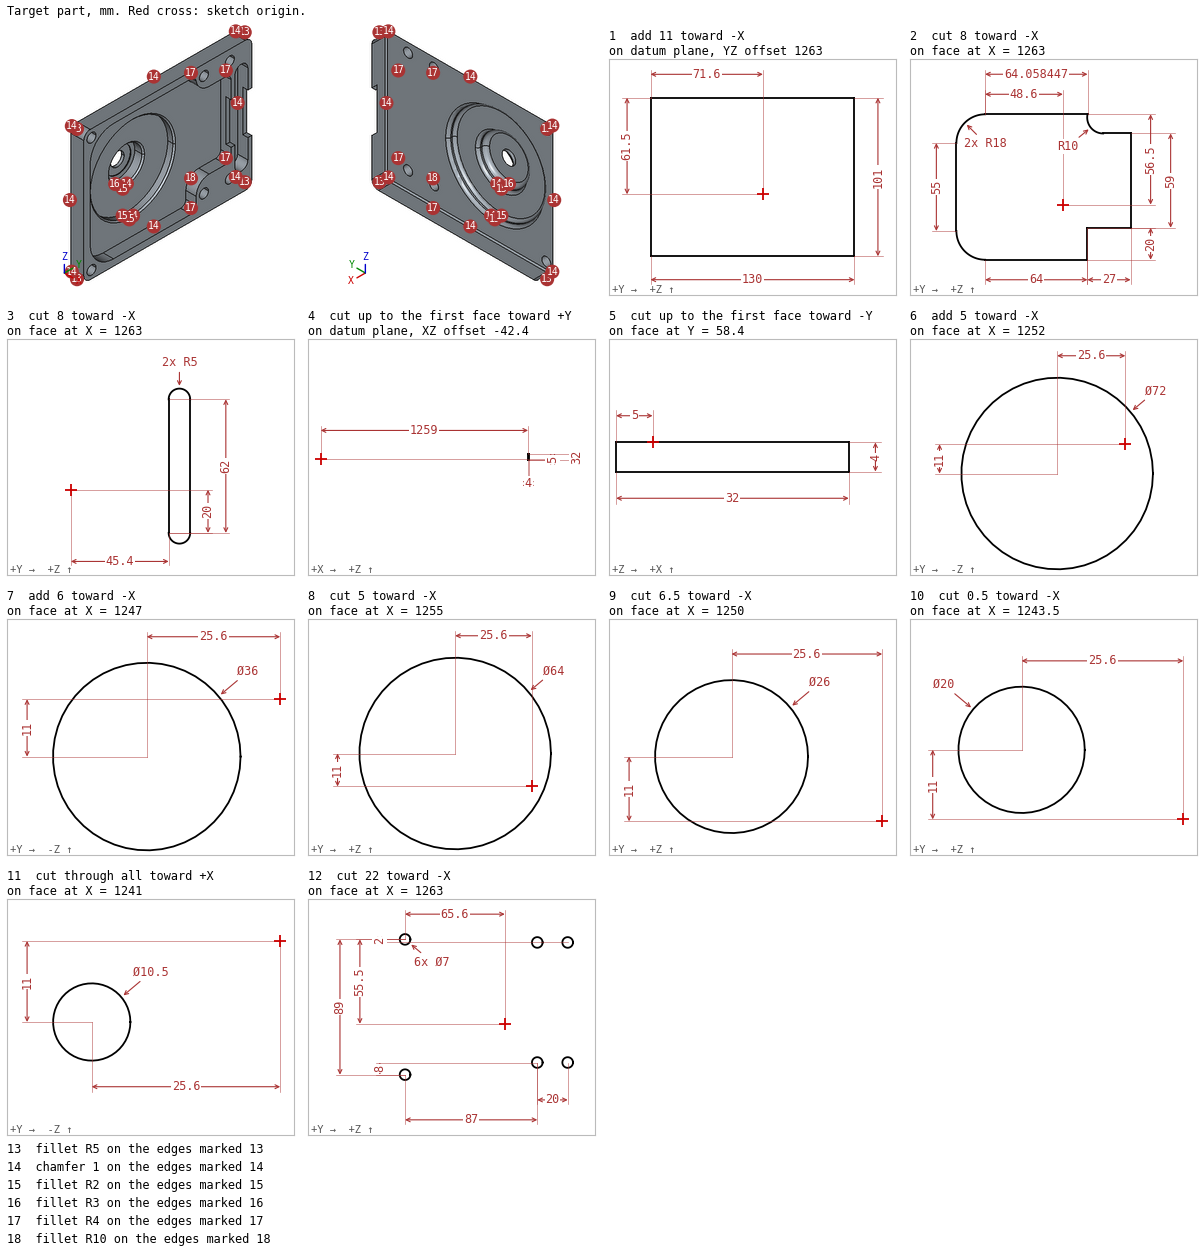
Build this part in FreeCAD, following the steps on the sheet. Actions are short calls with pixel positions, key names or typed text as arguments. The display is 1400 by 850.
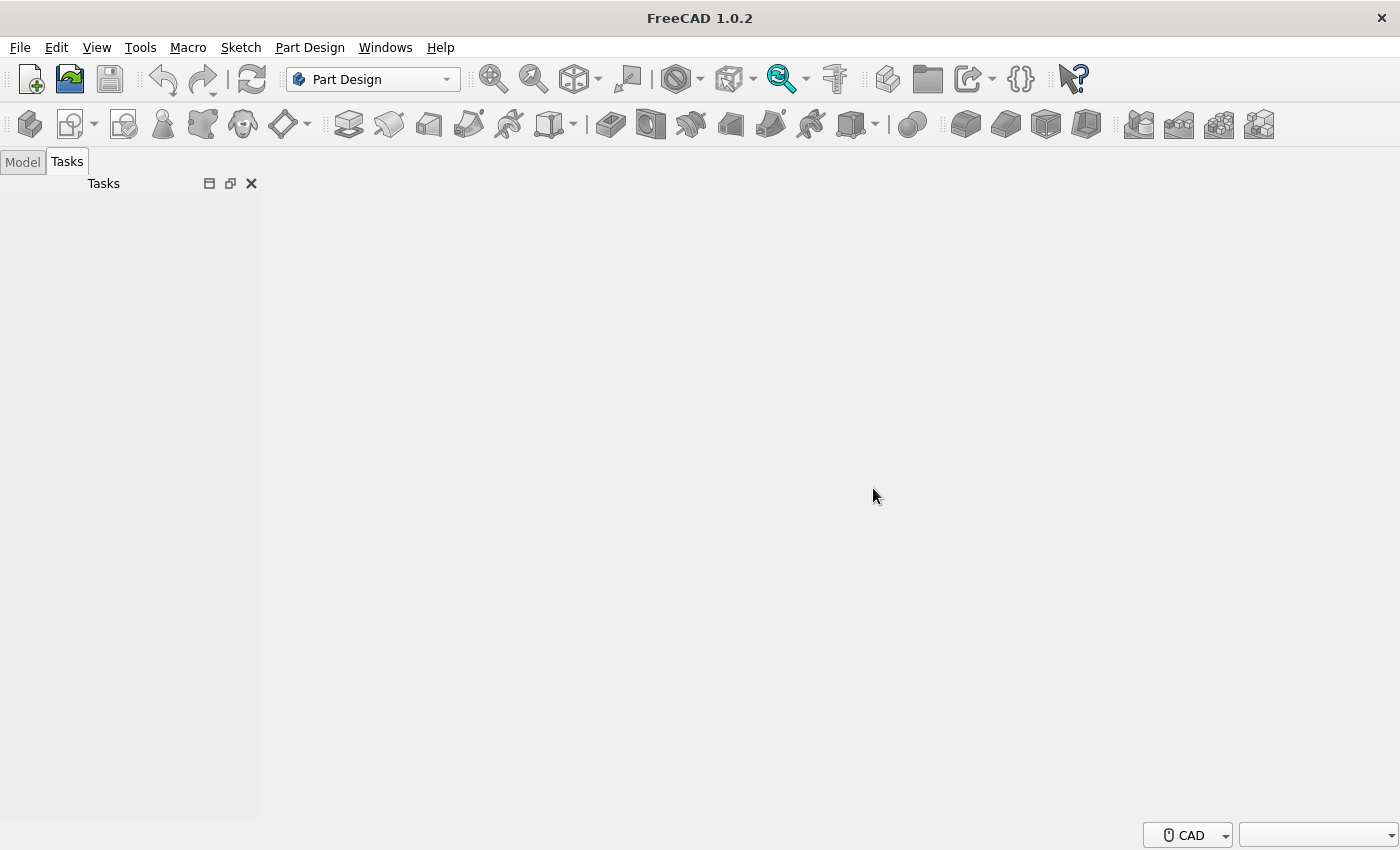
key(ctrl+n)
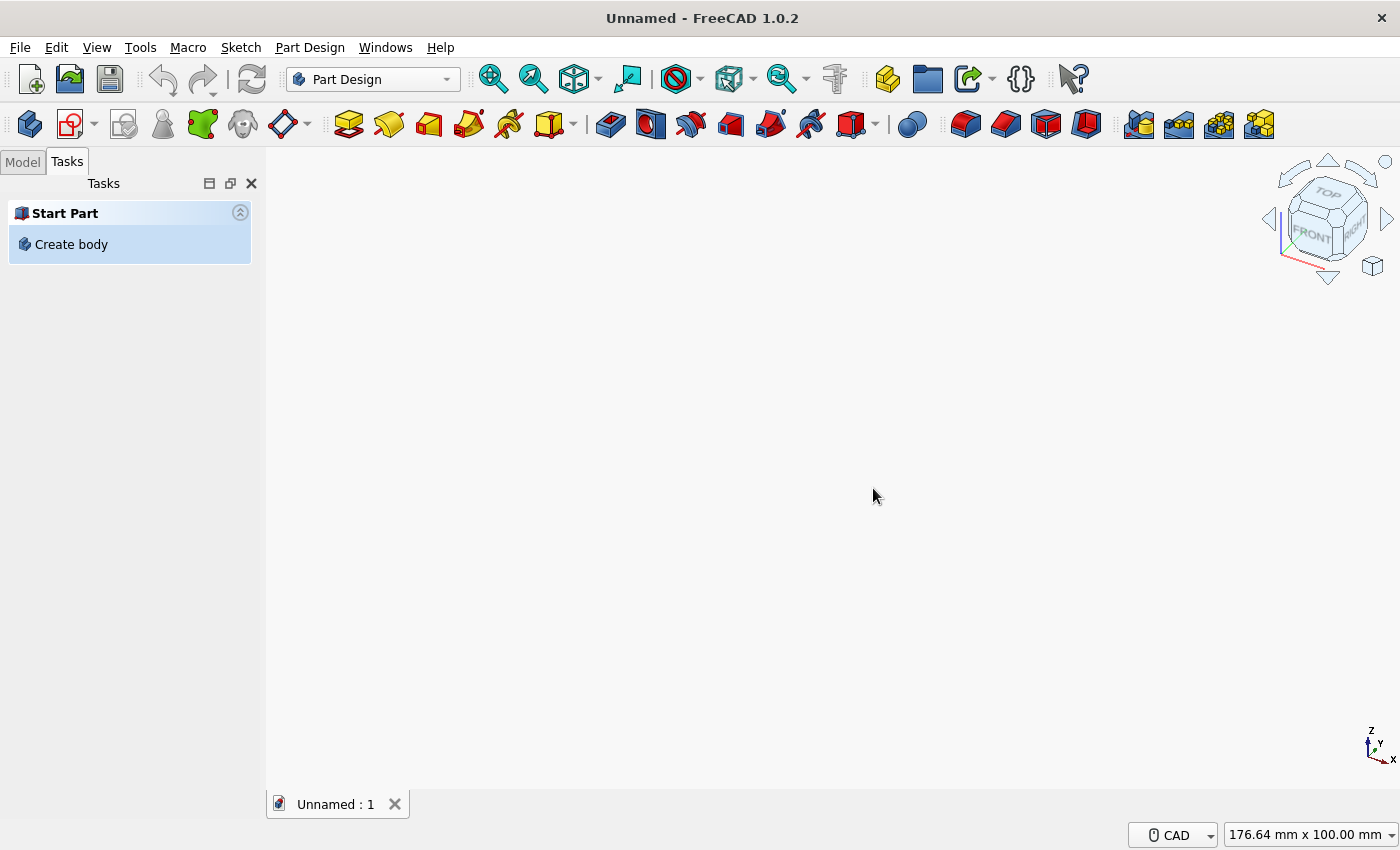
click(30, 124)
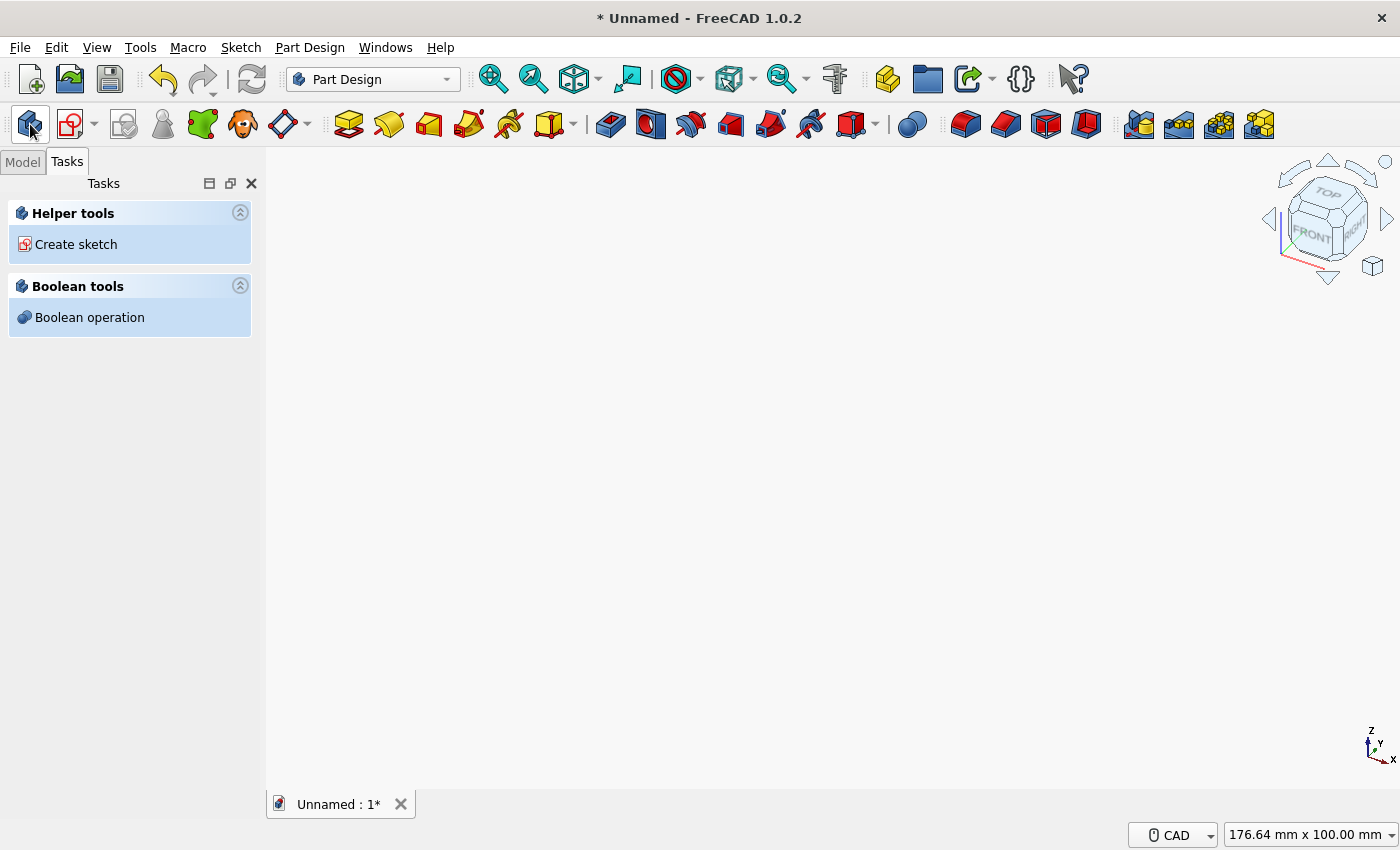
click(23, 161)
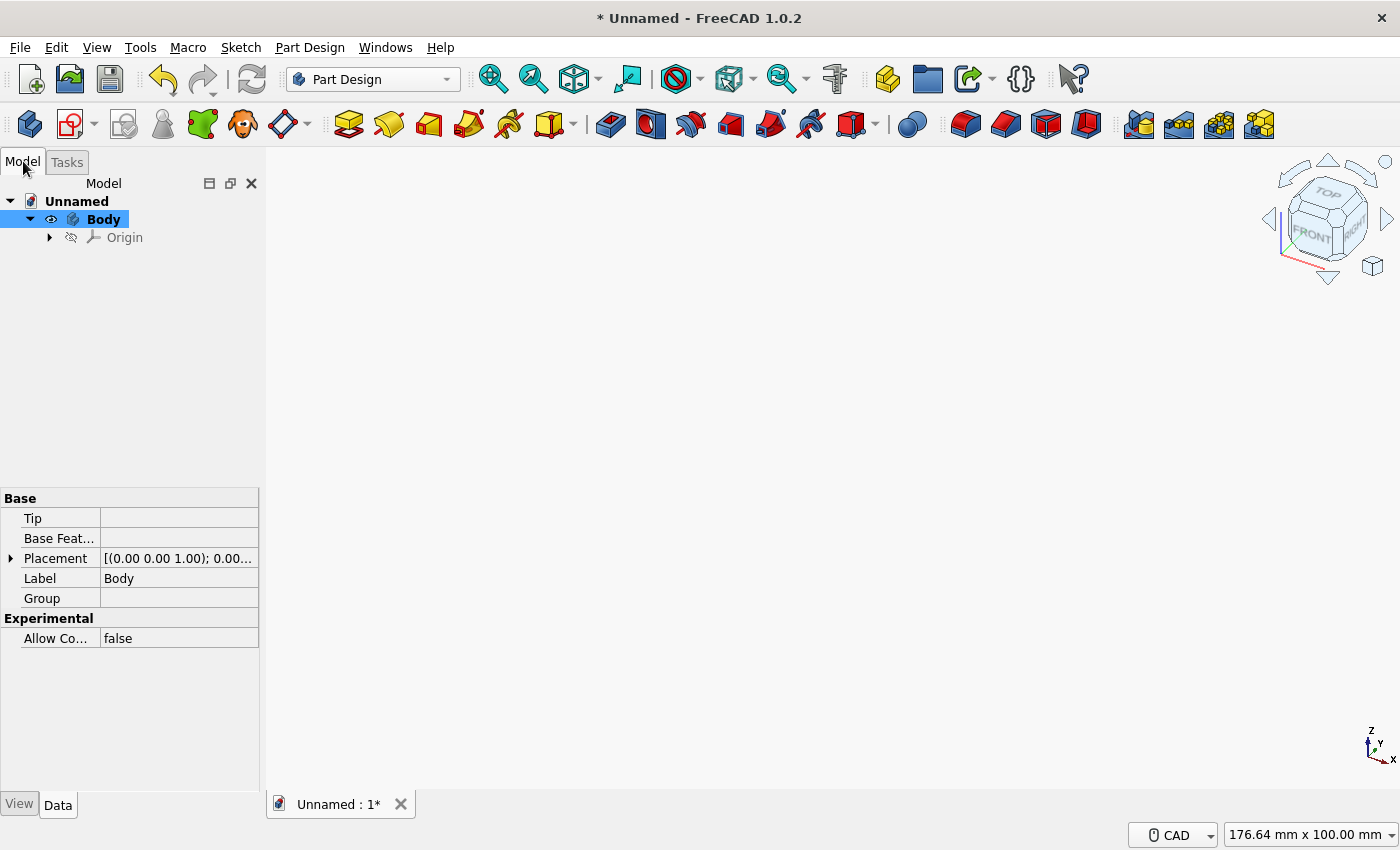
click(50, 237)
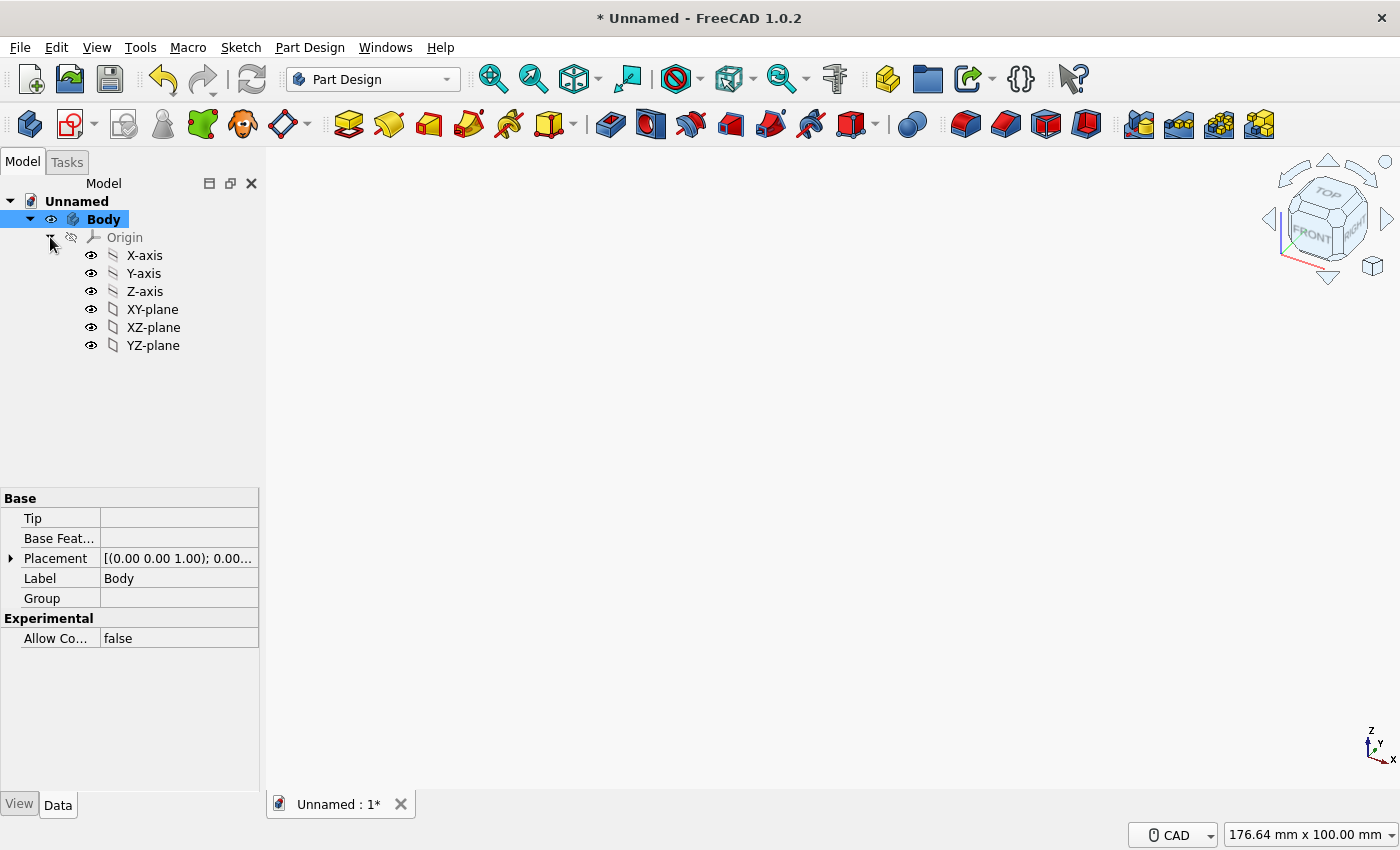
click(136, 345)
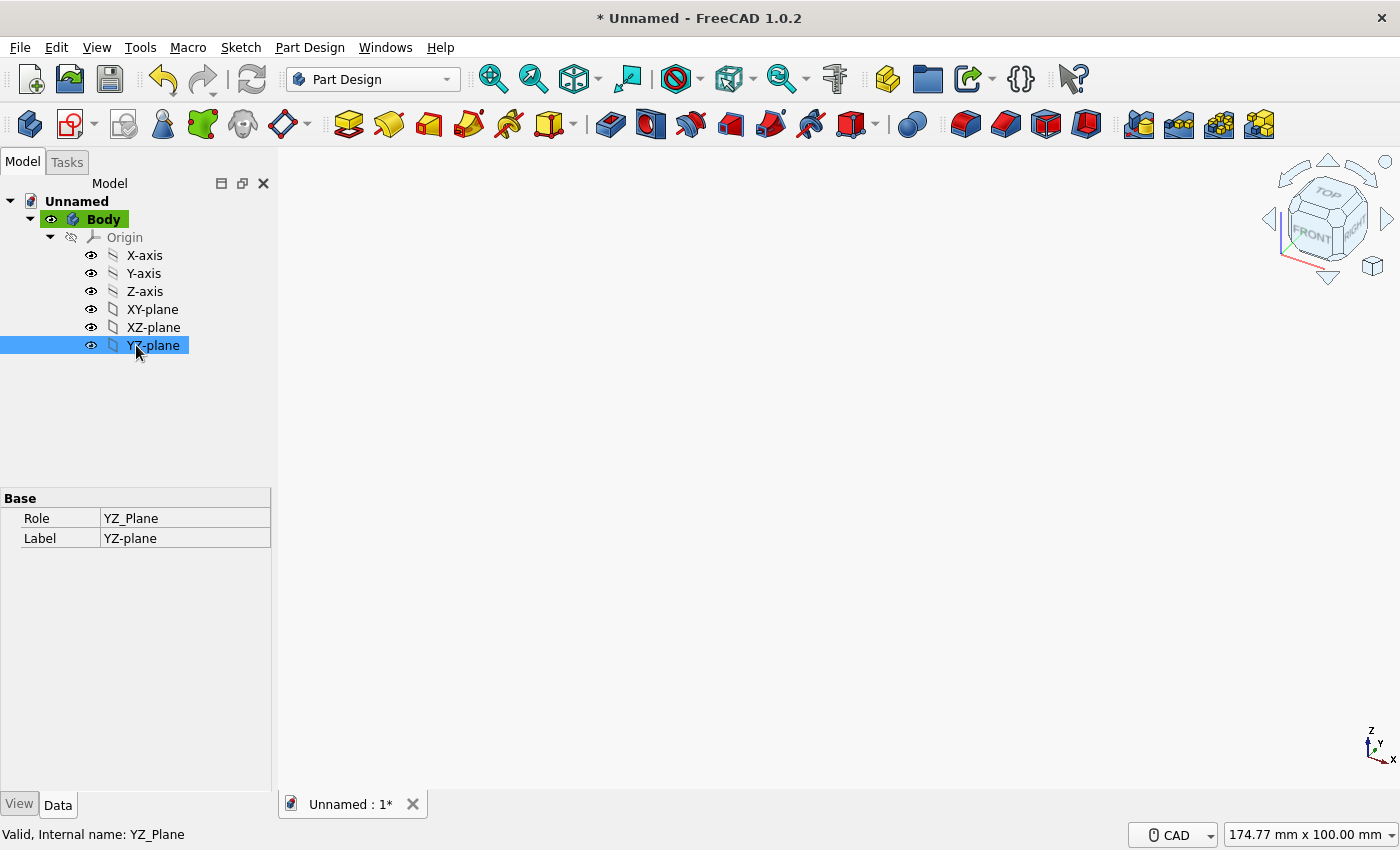
click(284, 124)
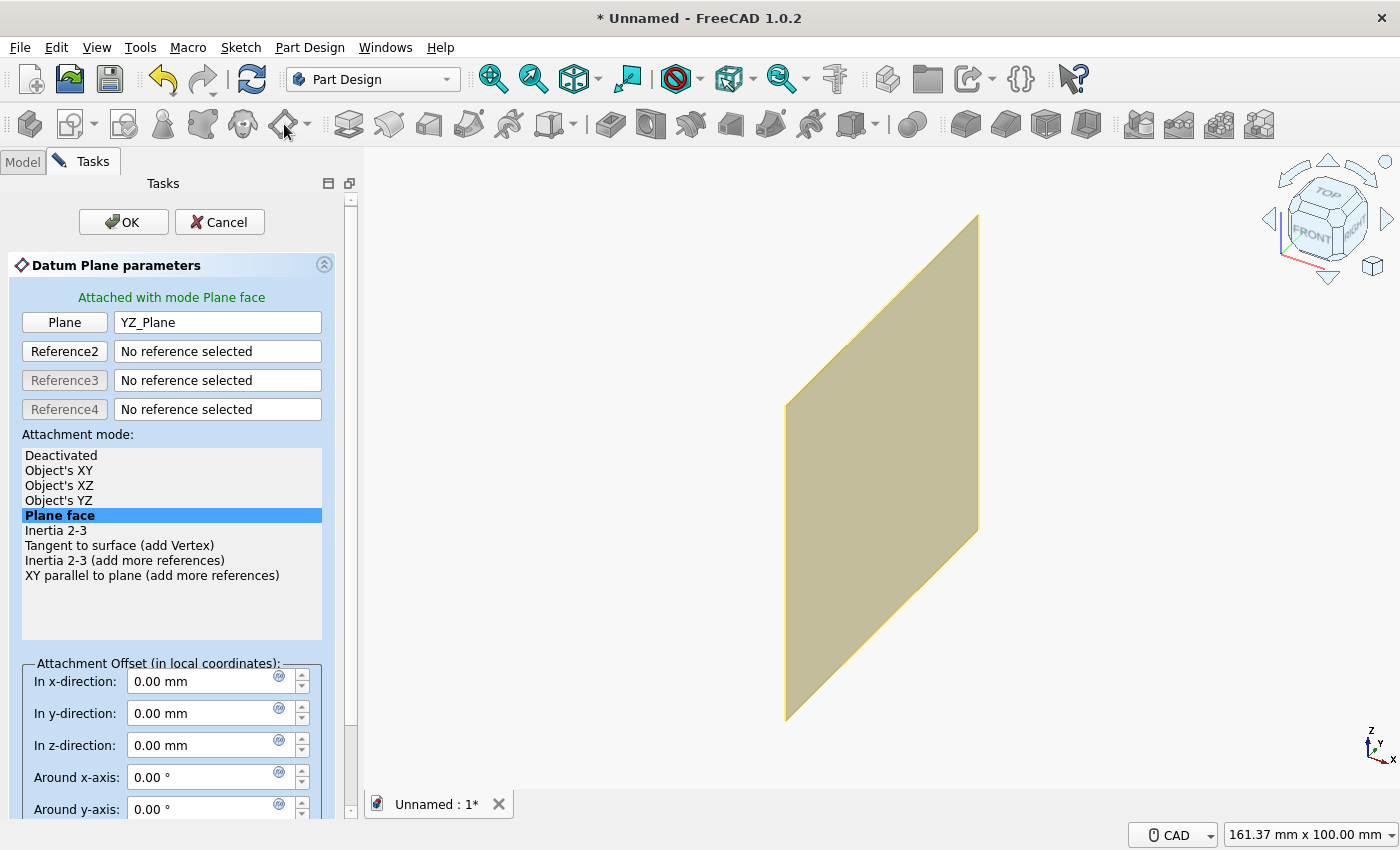
triple_click(210, 745)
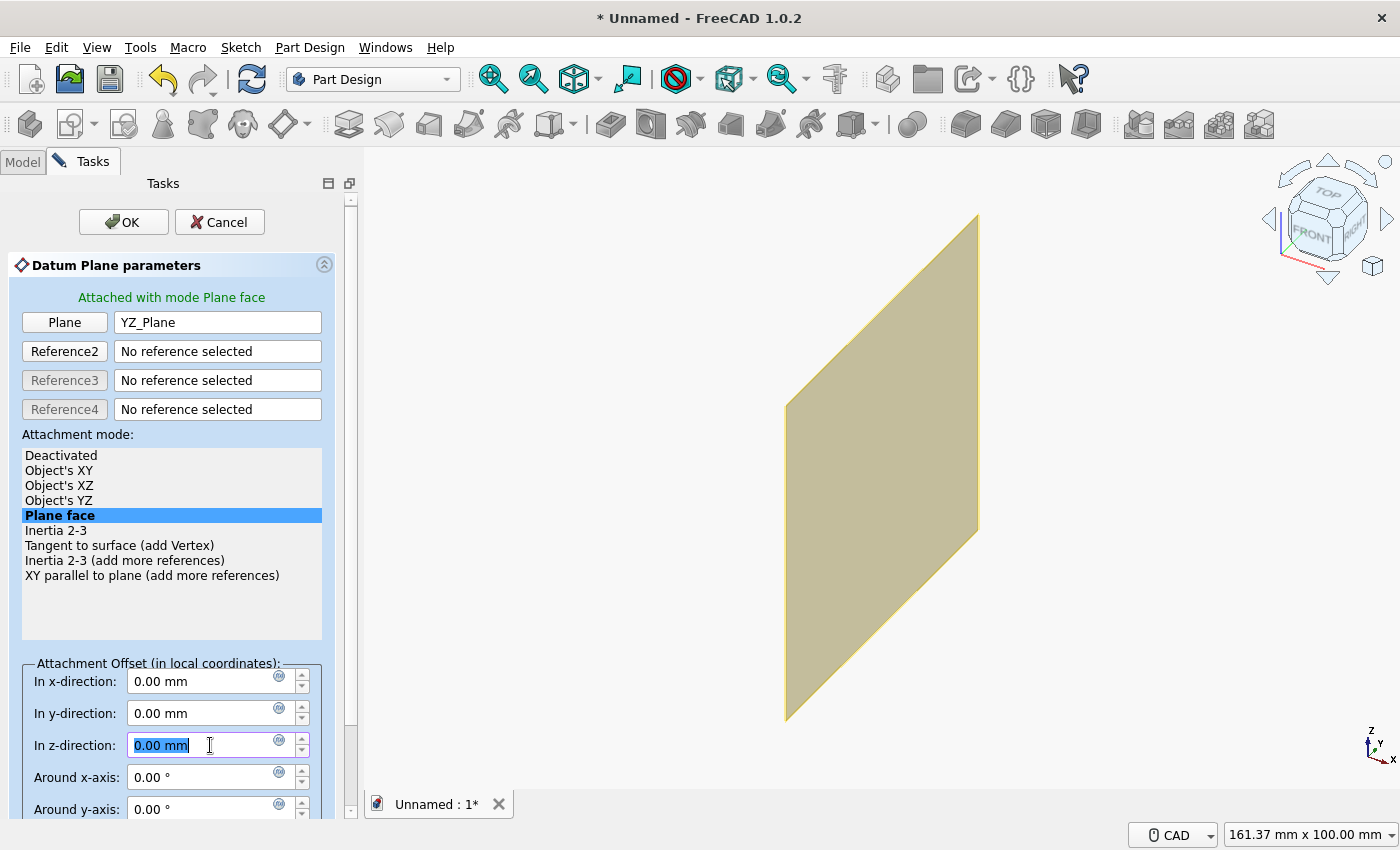
text(1263)
key(Tab)